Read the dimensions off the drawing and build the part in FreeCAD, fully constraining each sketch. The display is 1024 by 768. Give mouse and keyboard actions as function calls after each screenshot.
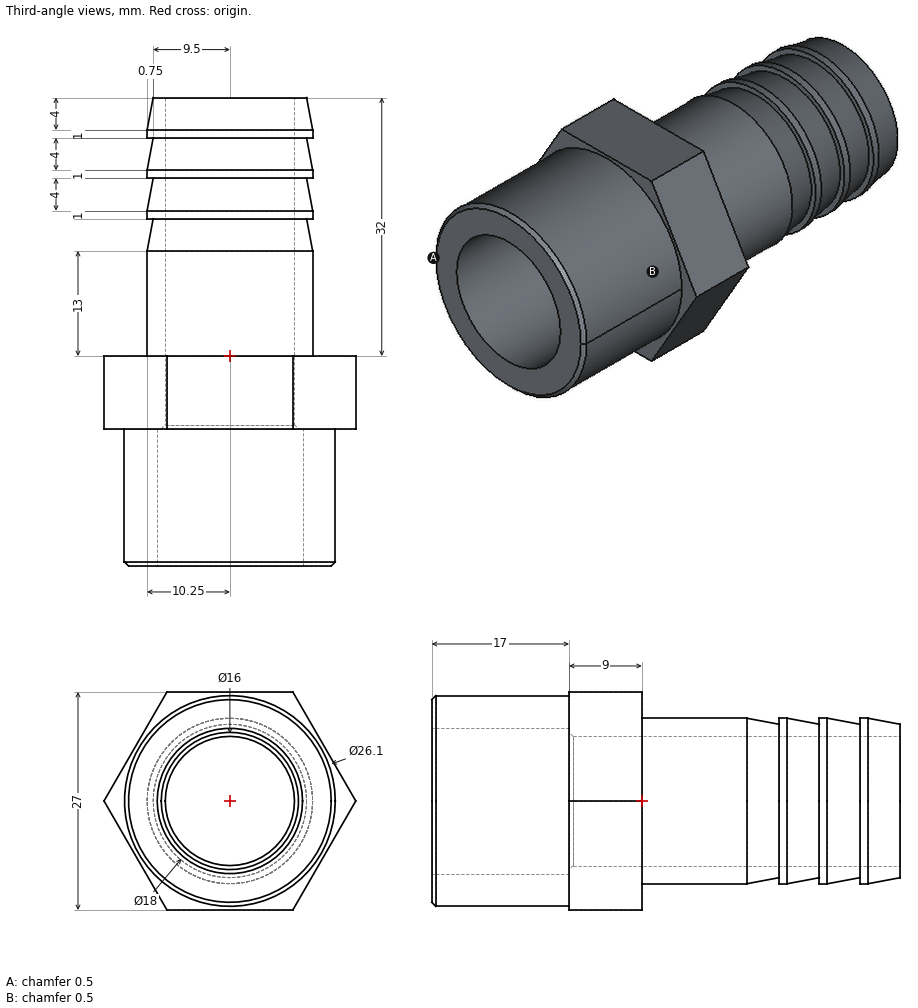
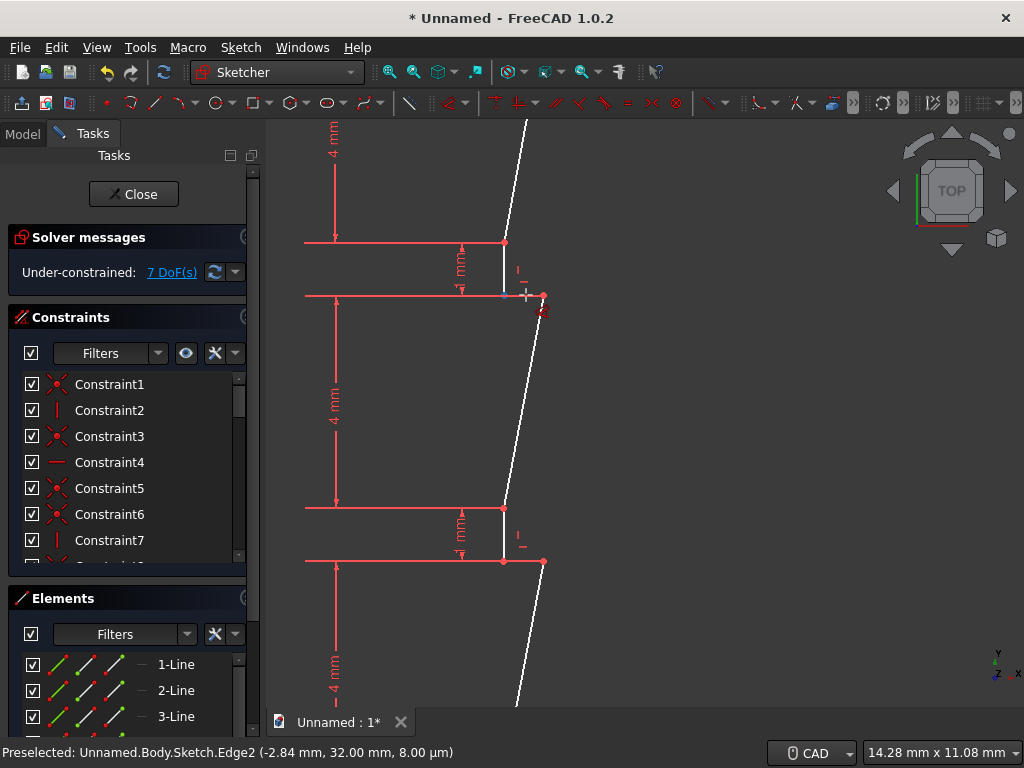
click(524, 296)
click(533, 262)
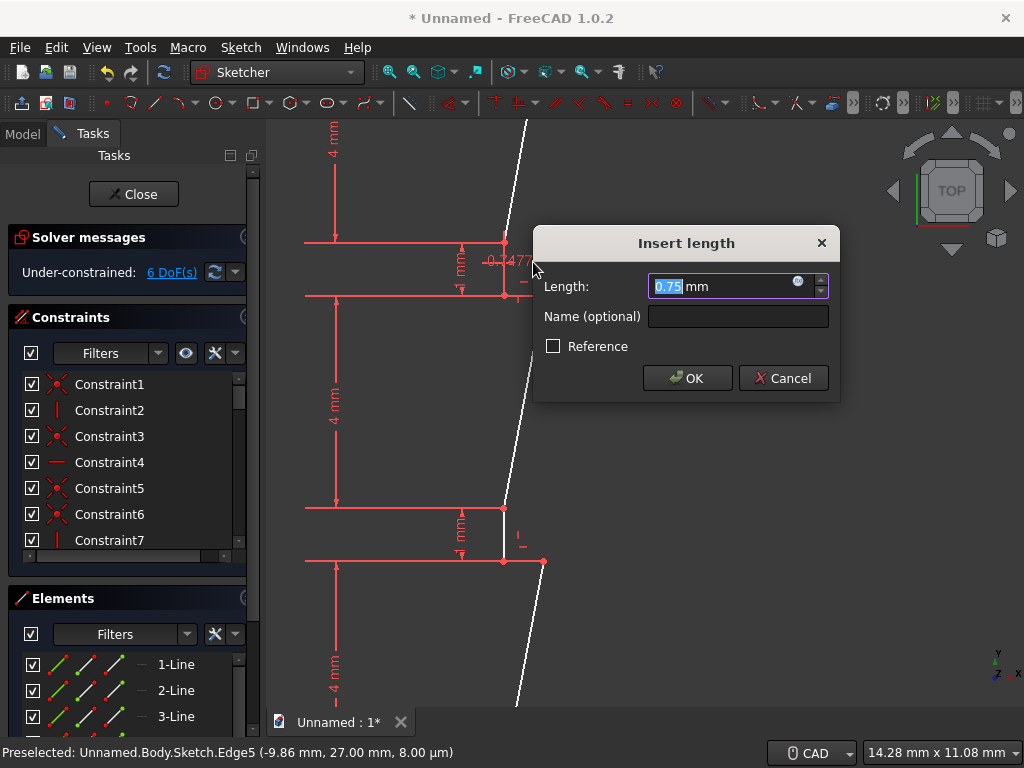
text(0.75)
key(Return)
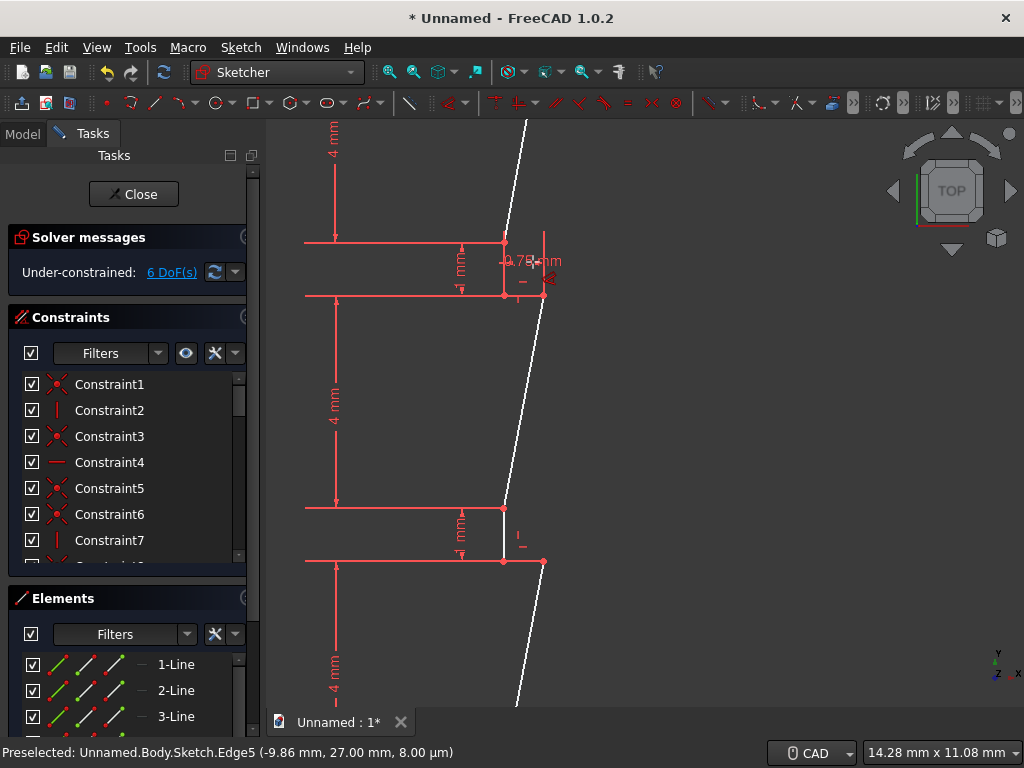
click(516, 561)
click(533, 527)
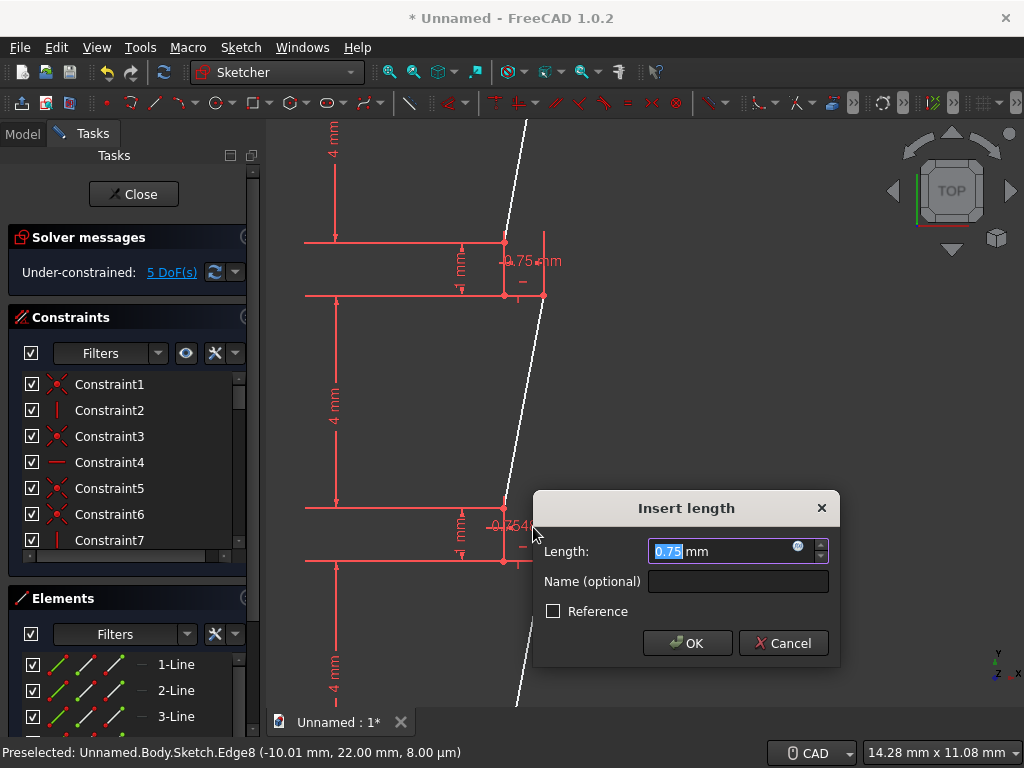
text(0.75)
key(Return)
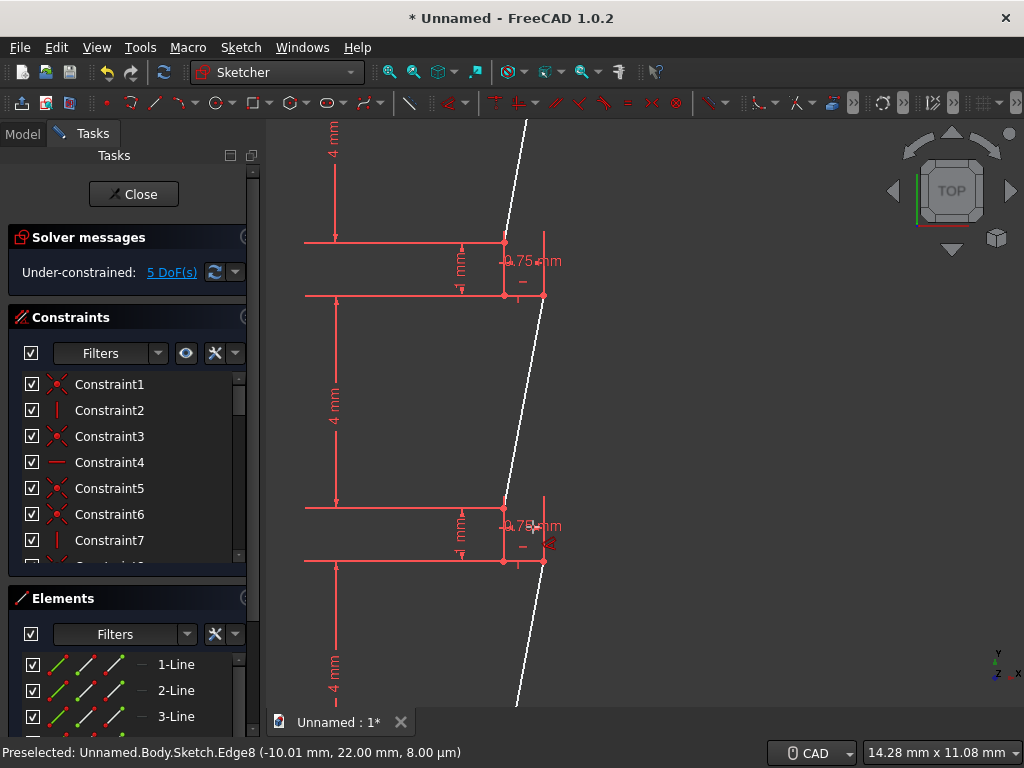
scroll(526, 295, down, 8)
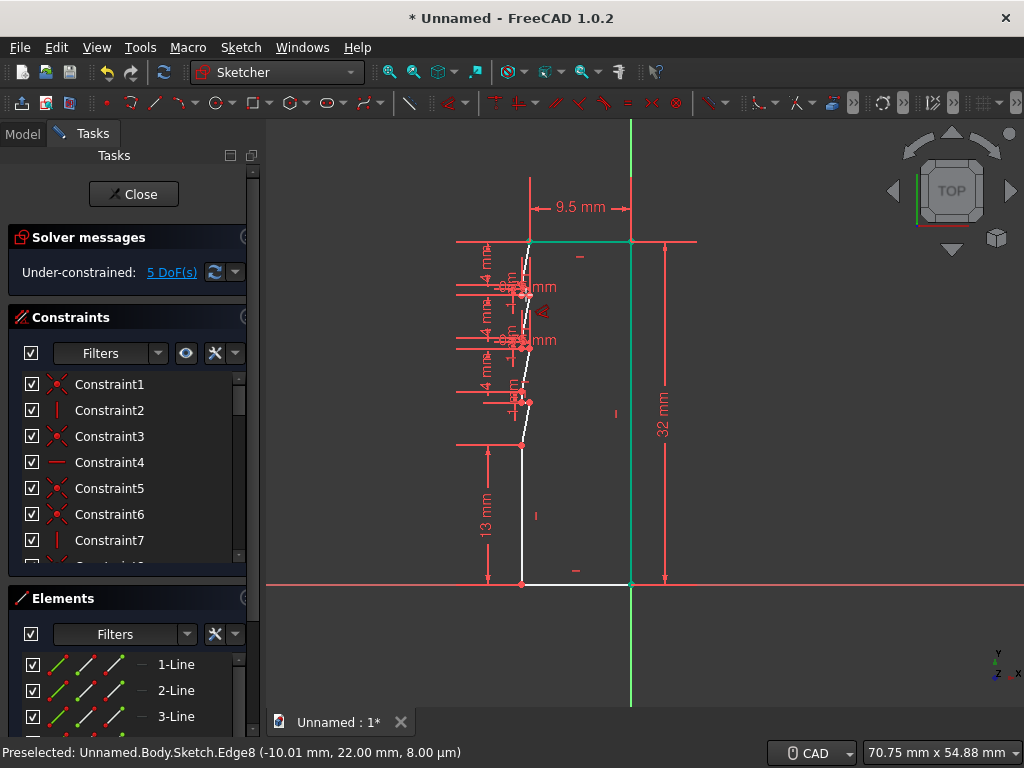
scroll(524, 403, up, 9)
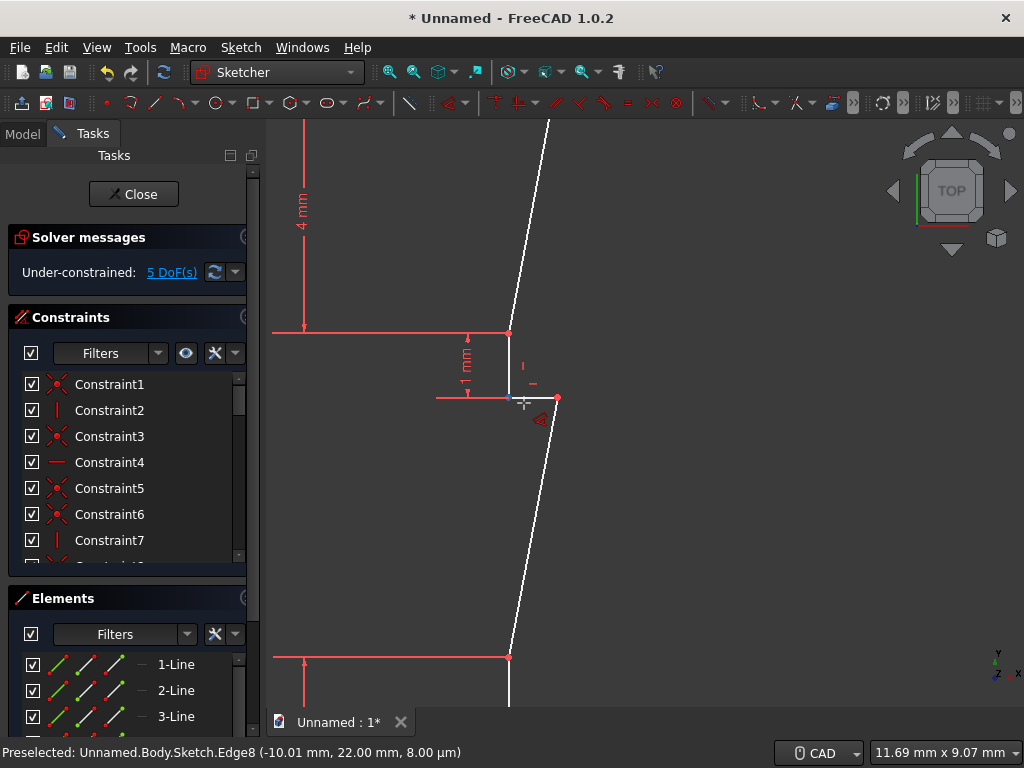
click(524, 398)
click(545, 364)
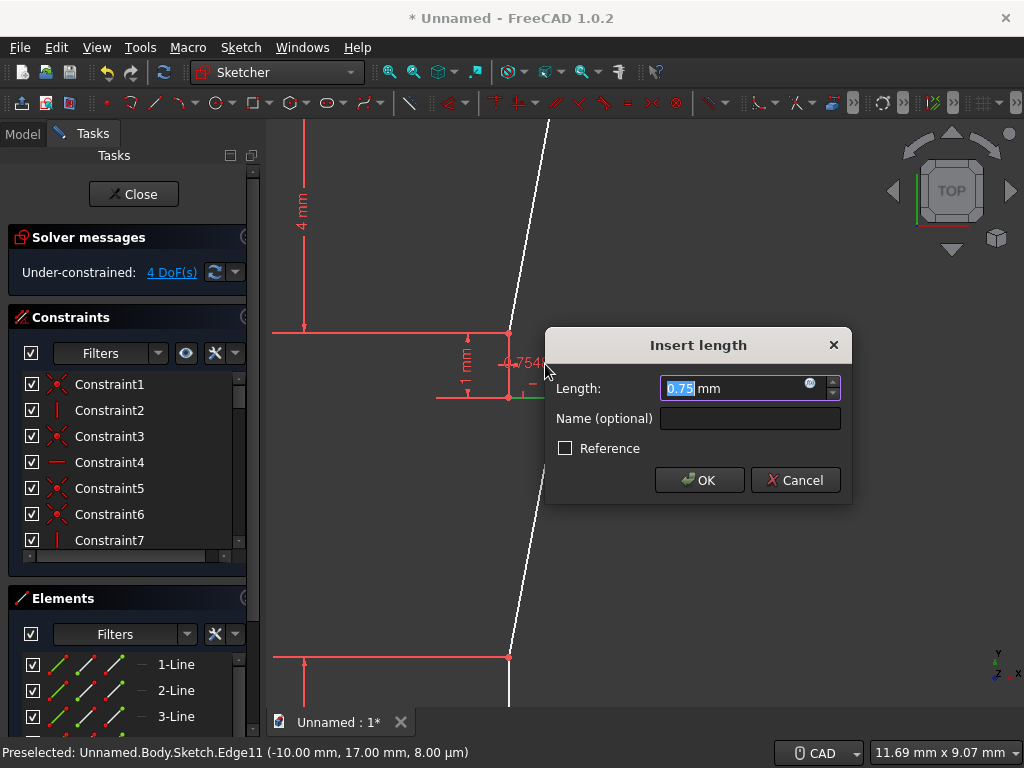
text(0.75)
key(Return)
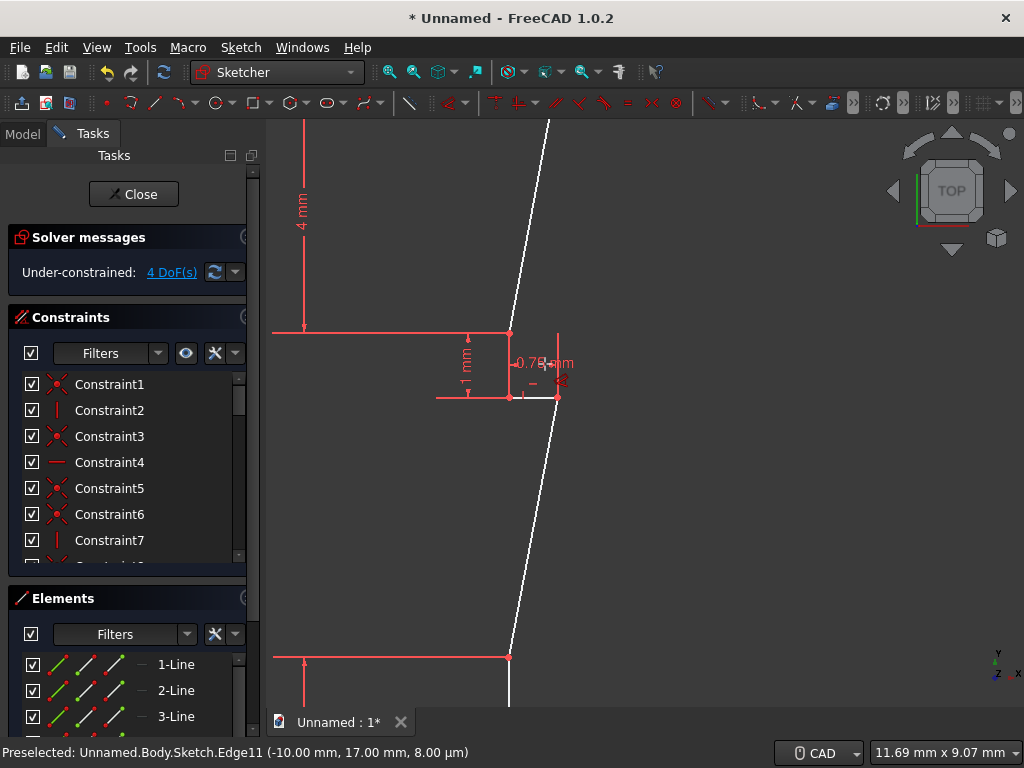
scroll(524, 403, down, 9)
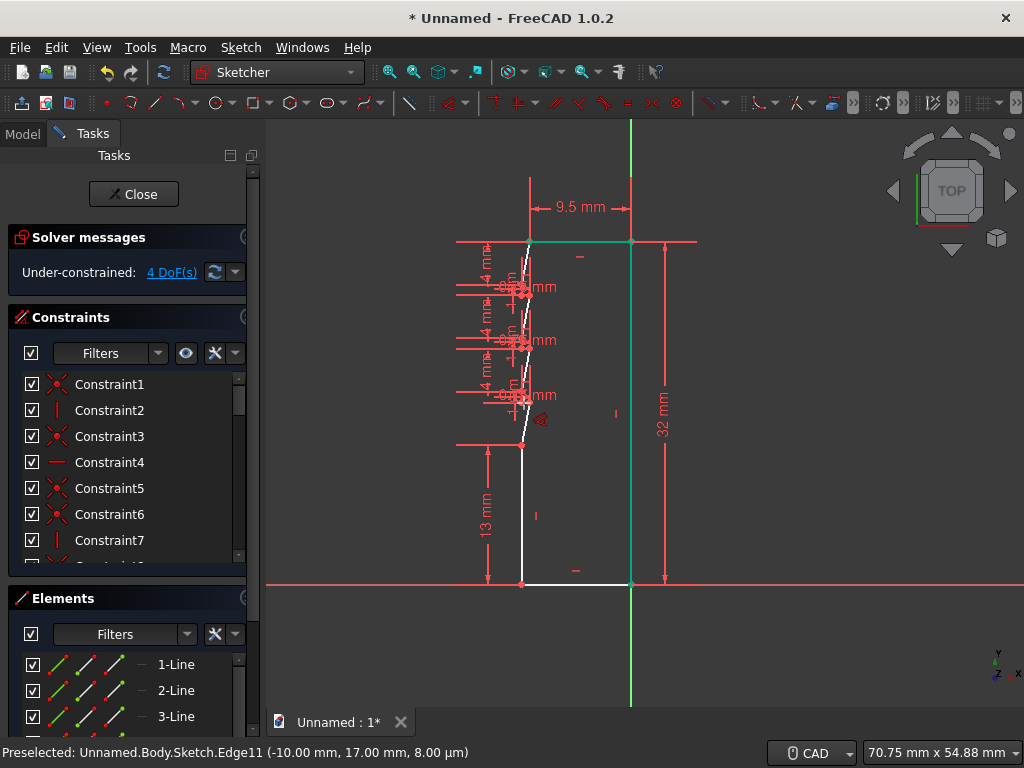
scroll(530, 295, up, 3)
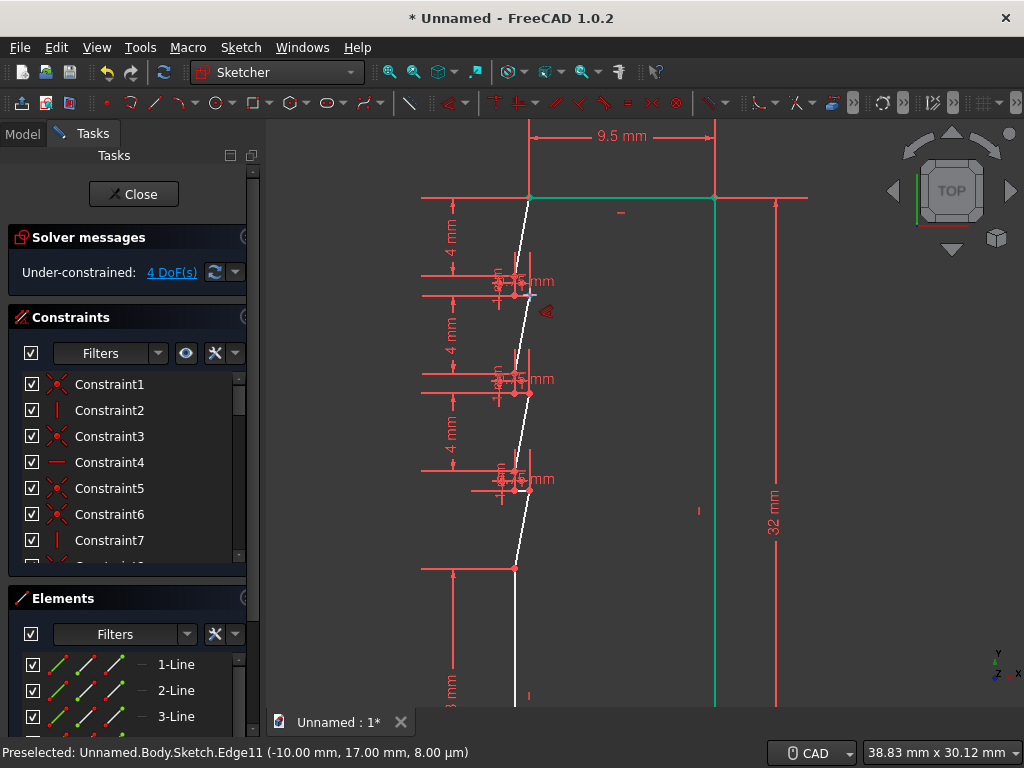
click(530, 296)
click(622, 262)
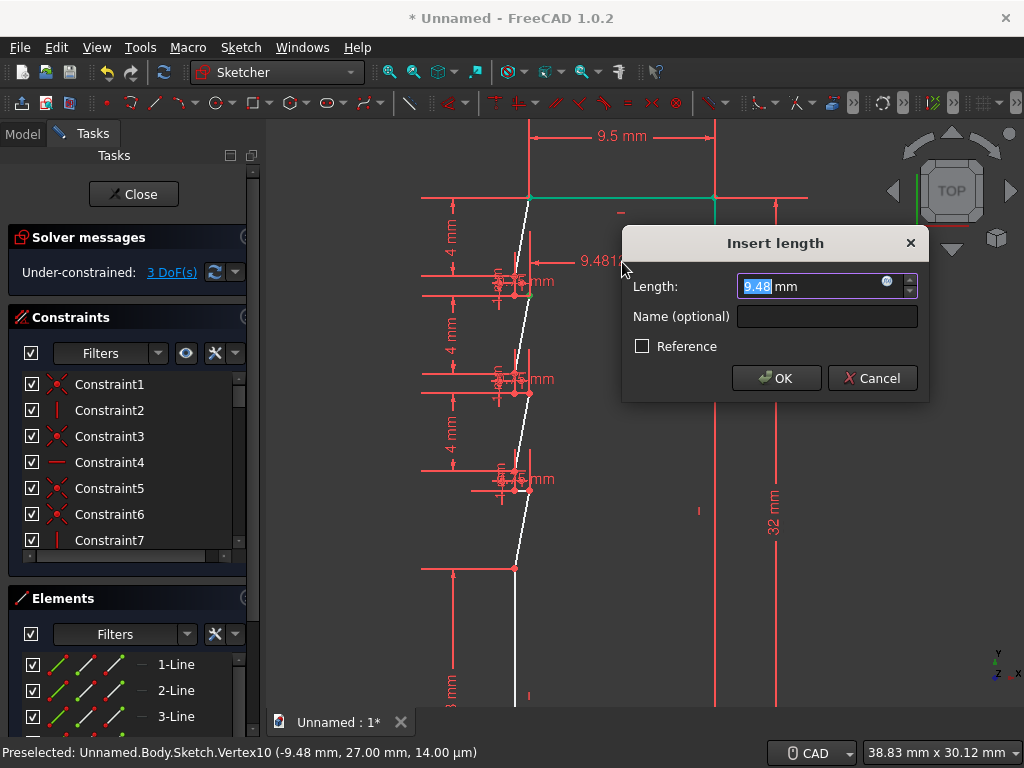
text(9.5)
key(Return)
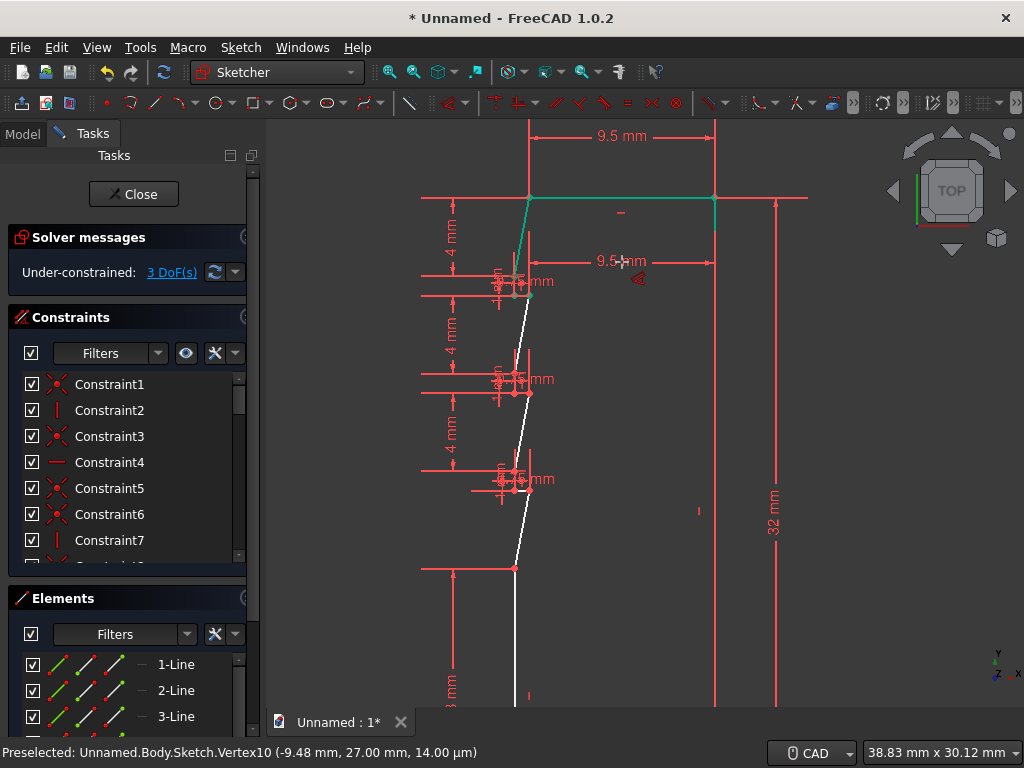
click(529, 393)
click(622, 359)